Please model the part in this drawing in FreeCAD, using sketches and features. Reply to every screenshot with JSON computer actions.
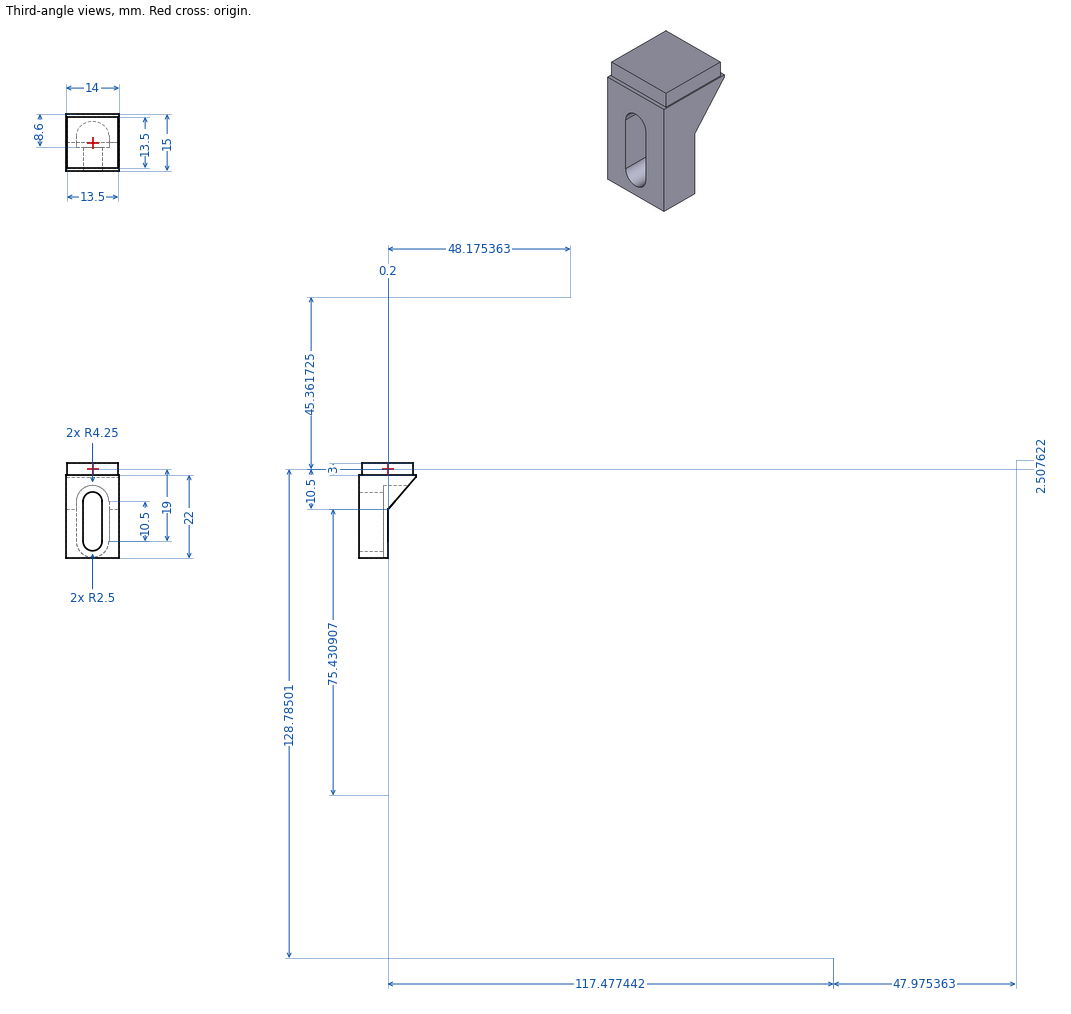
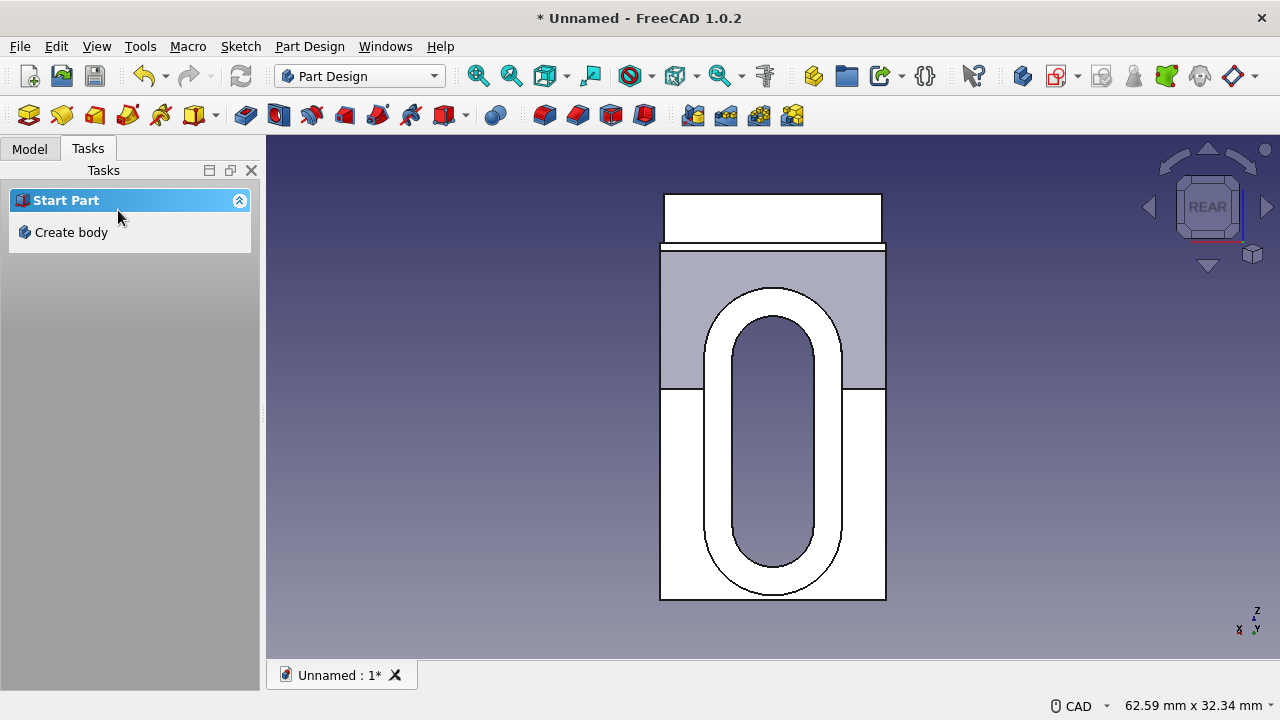
{"action": "key", "text": "0"}